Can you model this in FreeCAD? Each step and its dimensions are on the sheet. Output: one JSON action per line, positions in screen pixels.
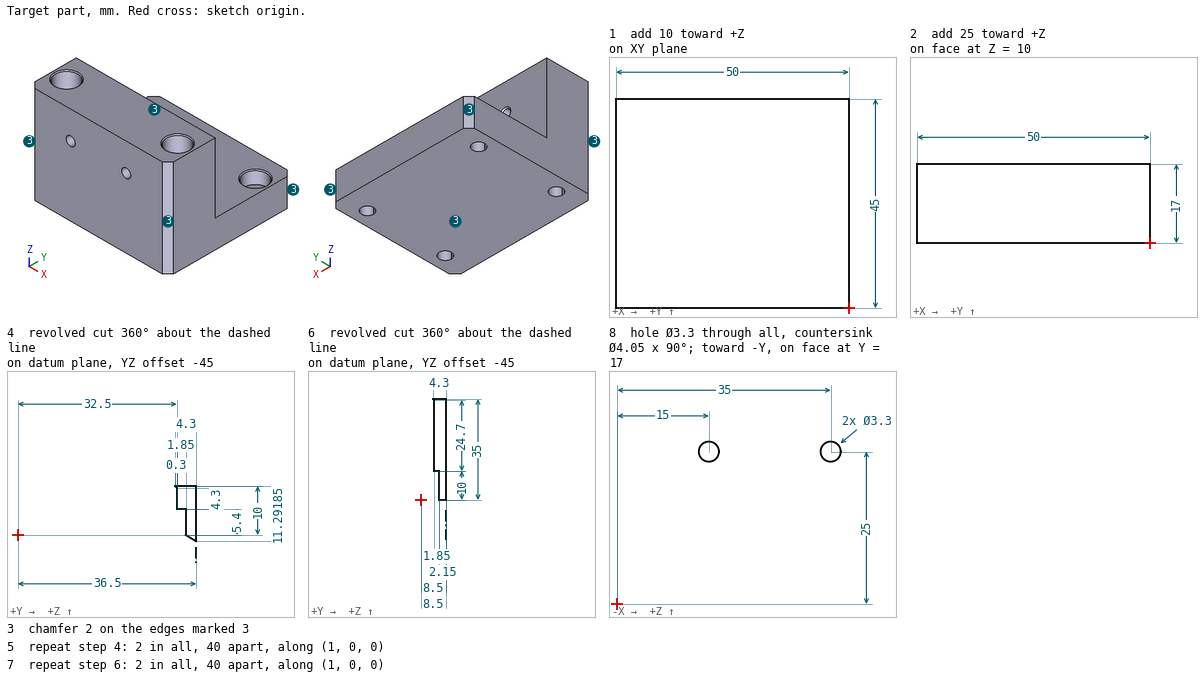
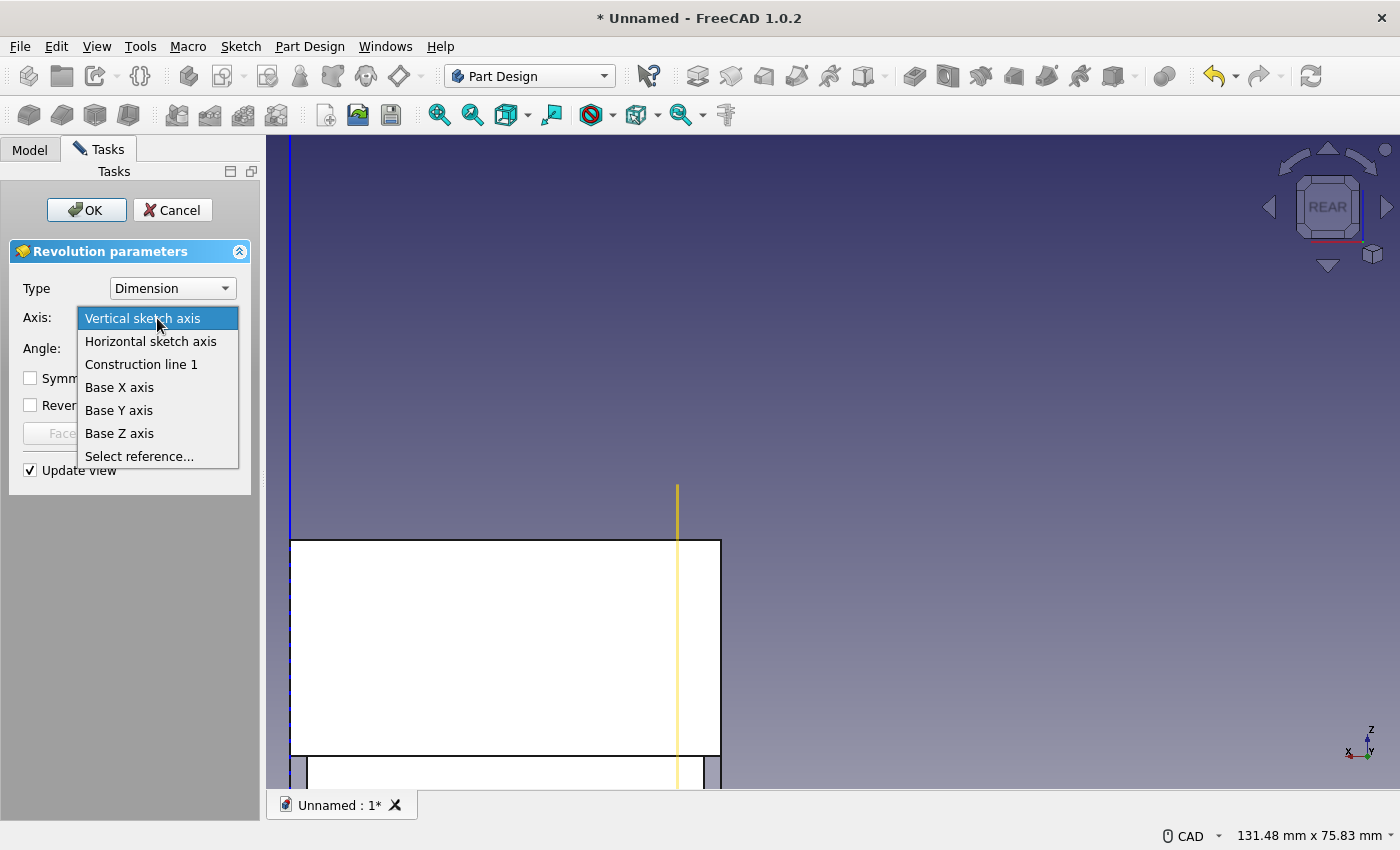
{"action": "left_click", "coordinate": [156, 364]}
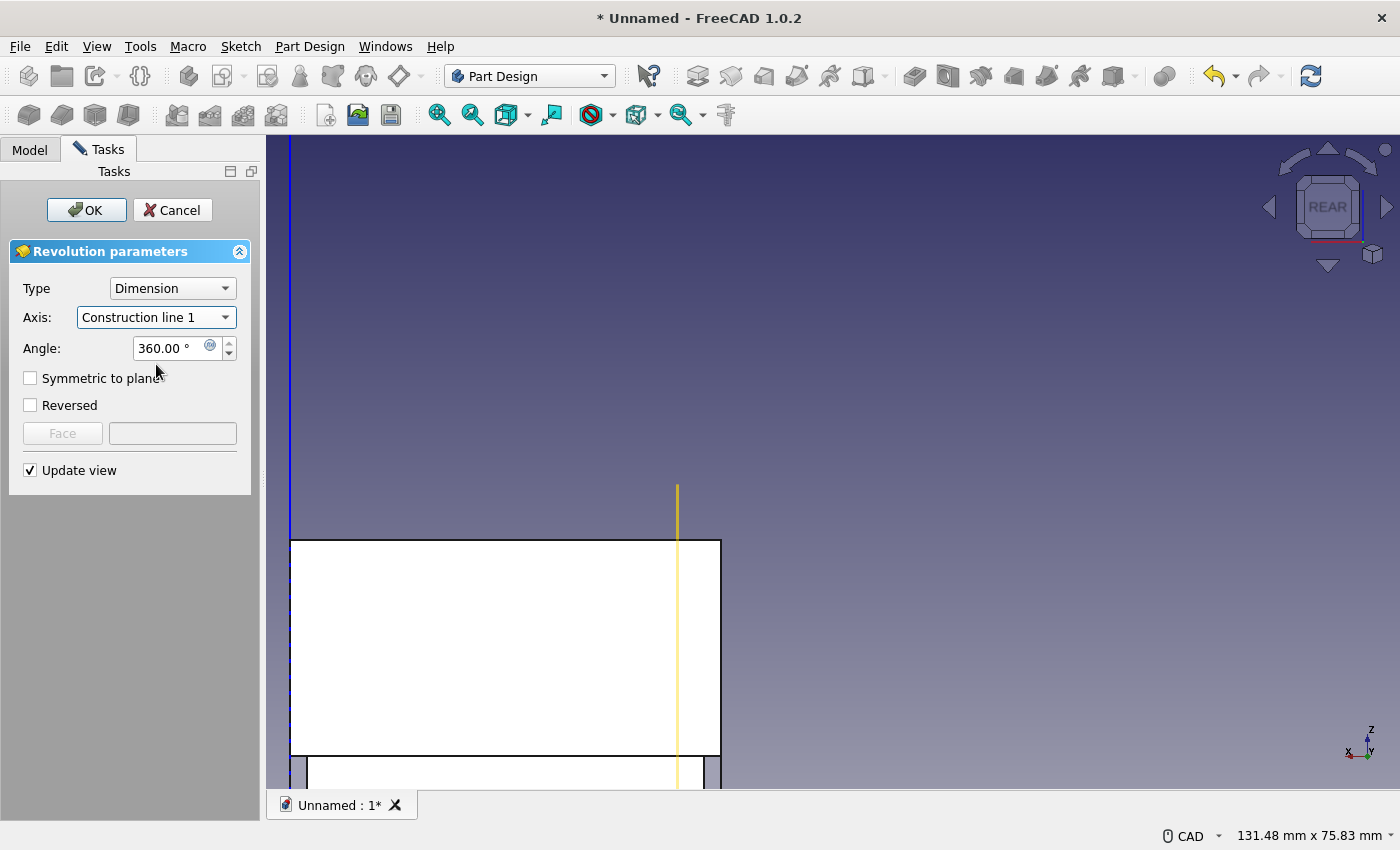
{"action": "left_click", "coordinate": [87, 210]}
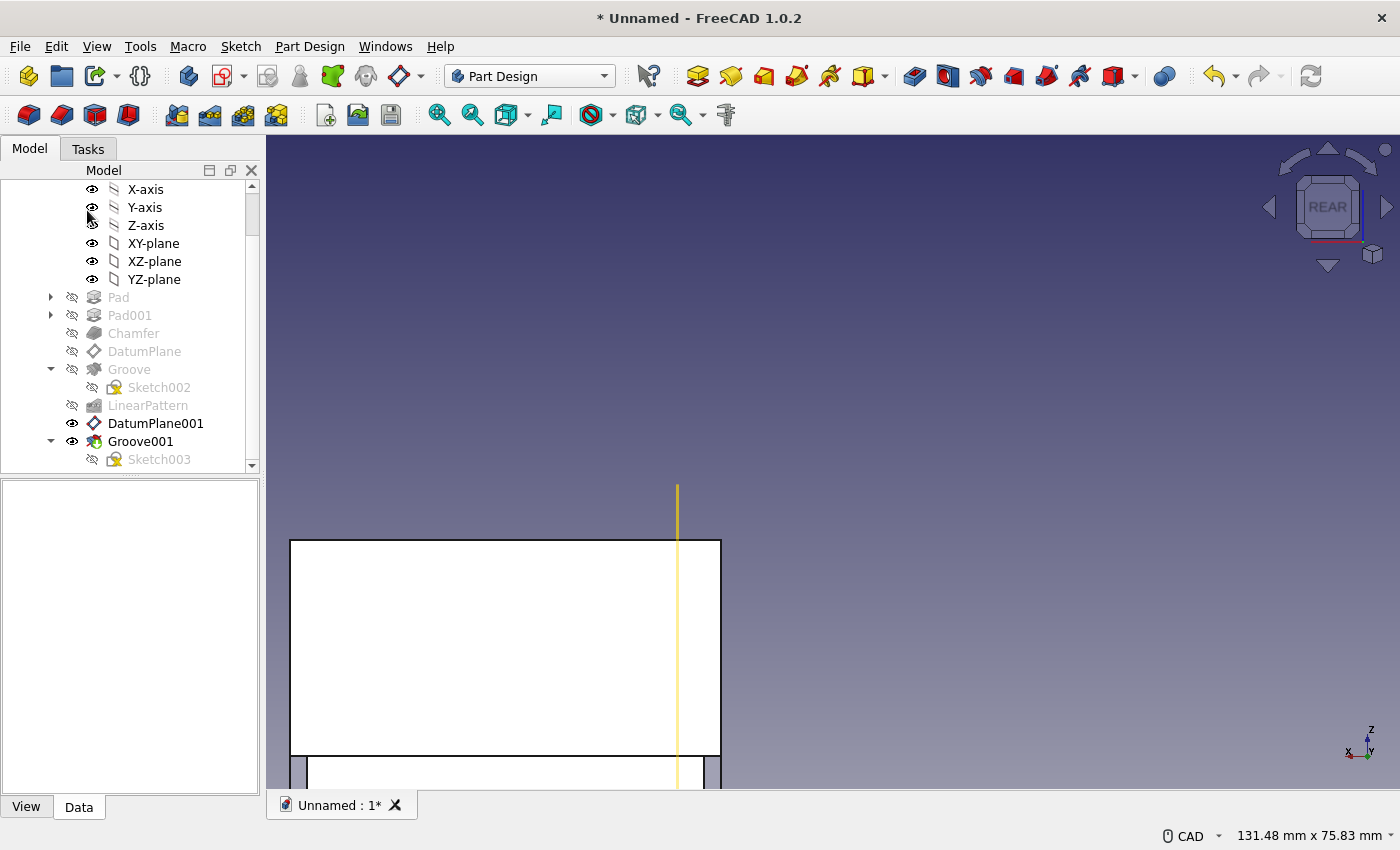
{"action": "left_click", "coordinate": [117, 423]}
{"action": "key", "text": "space"}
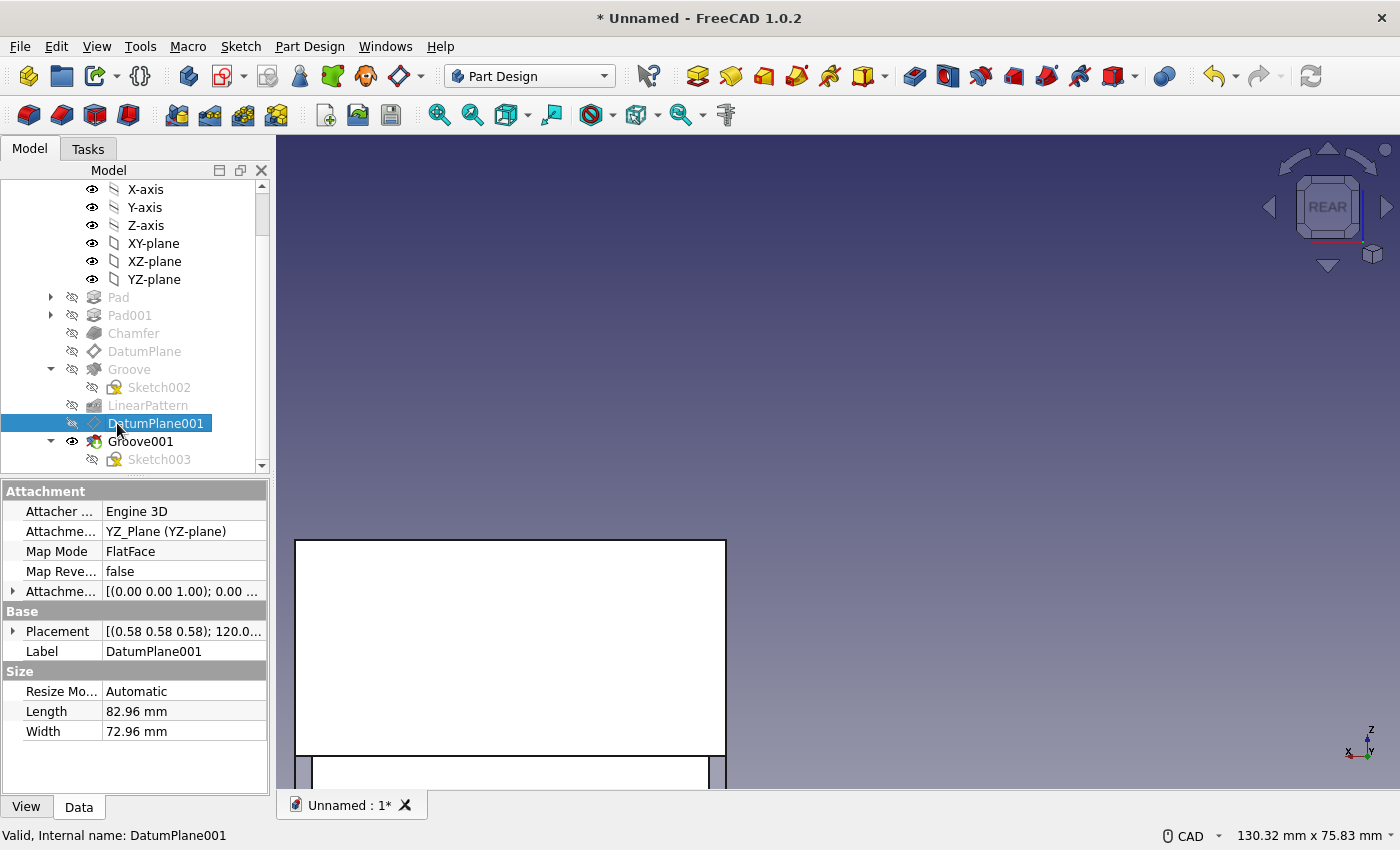
{"action": "left_click", "coordinate": [440, 116]}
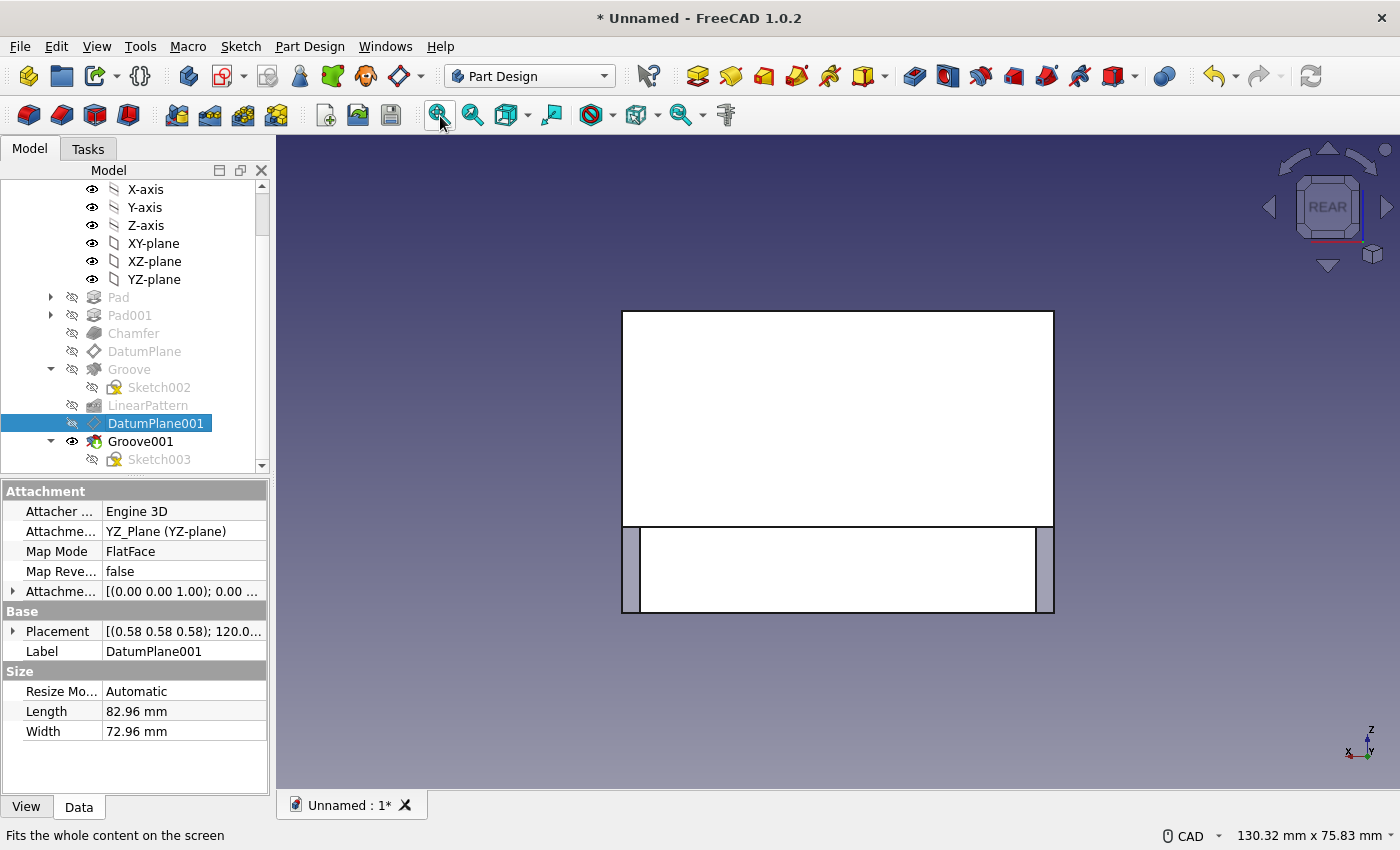
{"action": "left_click", "coordinate": [117, 441]}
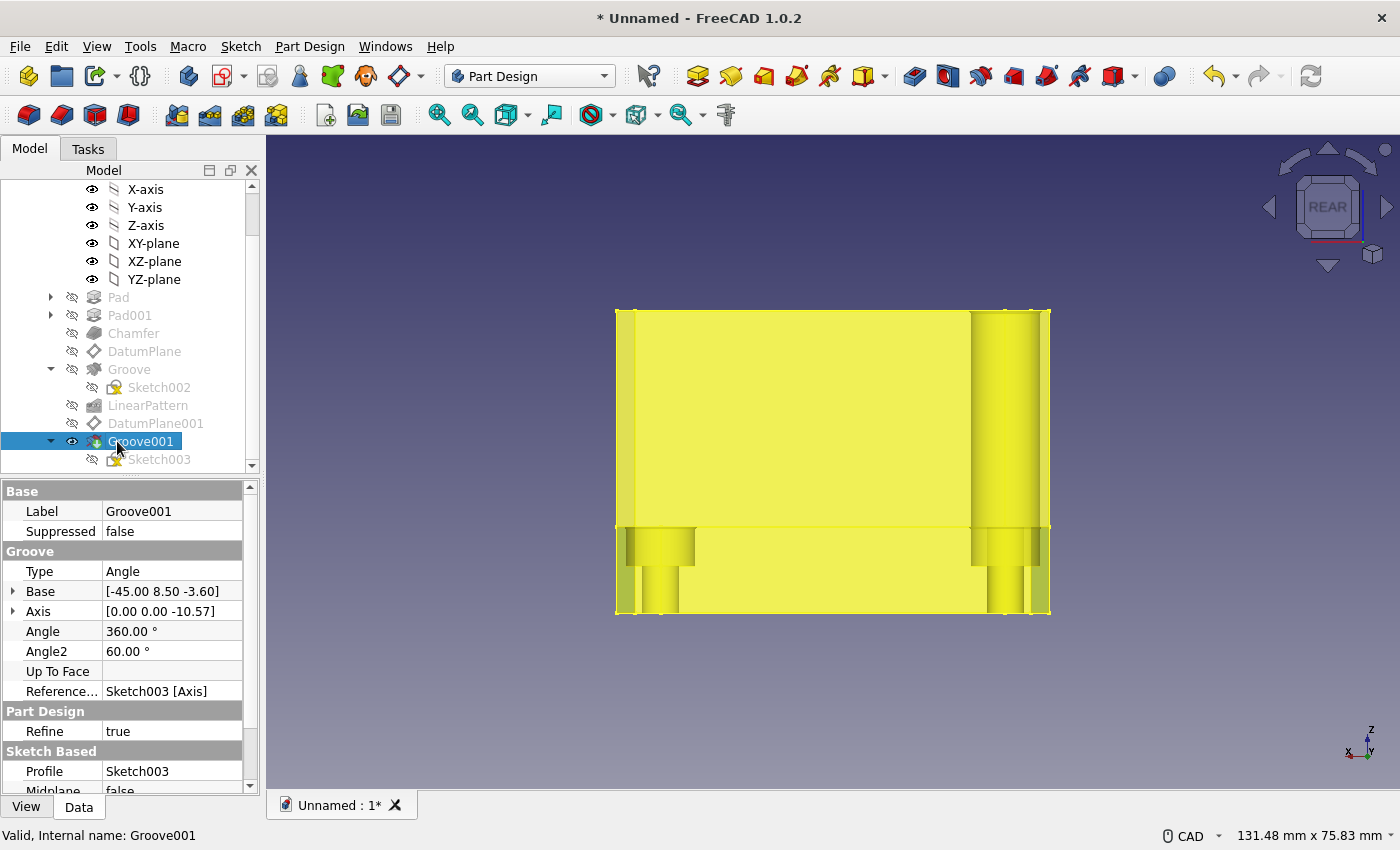
{"action": "left_click", "coordinate": [210, 116]}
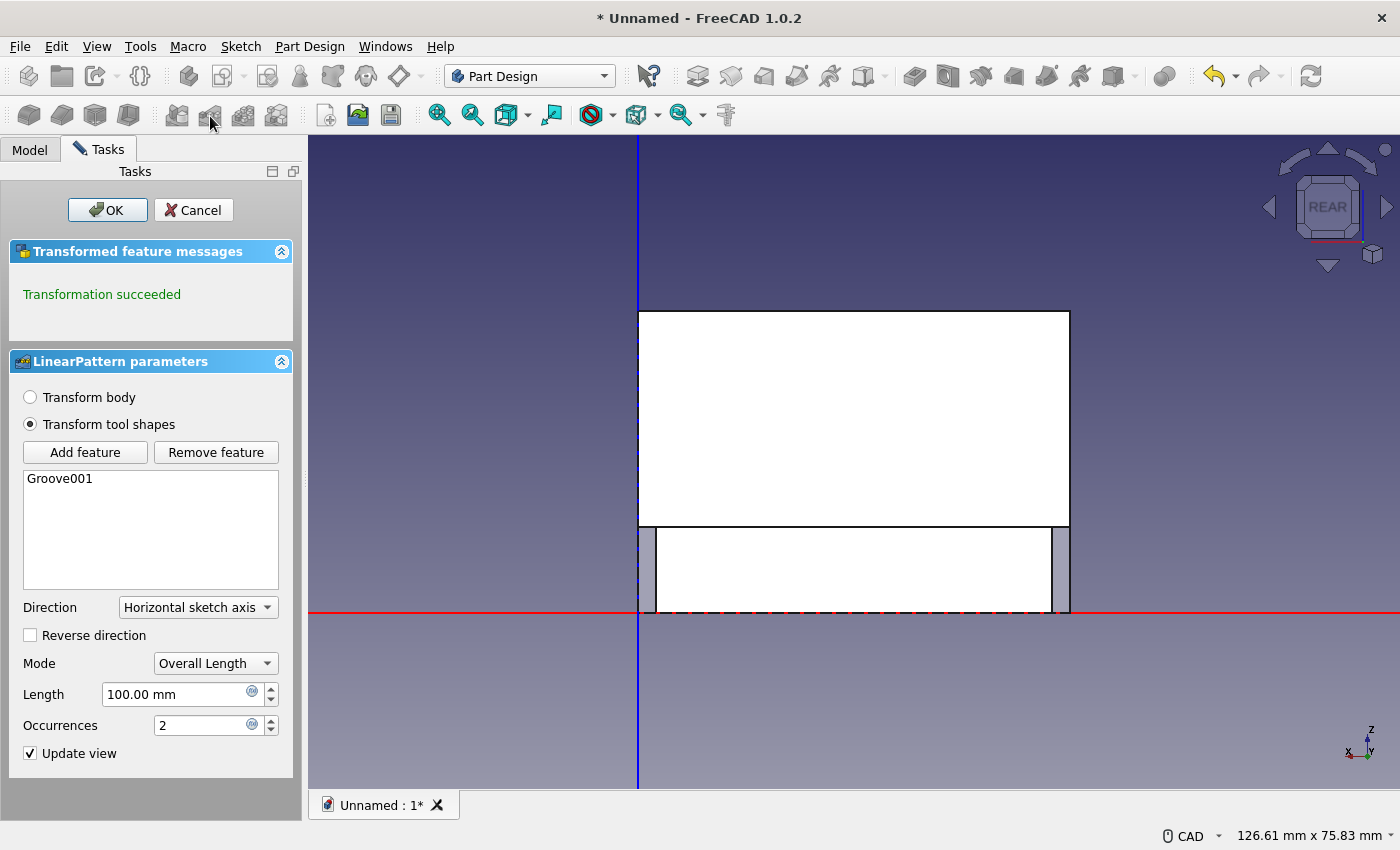
{"action": "left_click", "coordinate": [199, 608]}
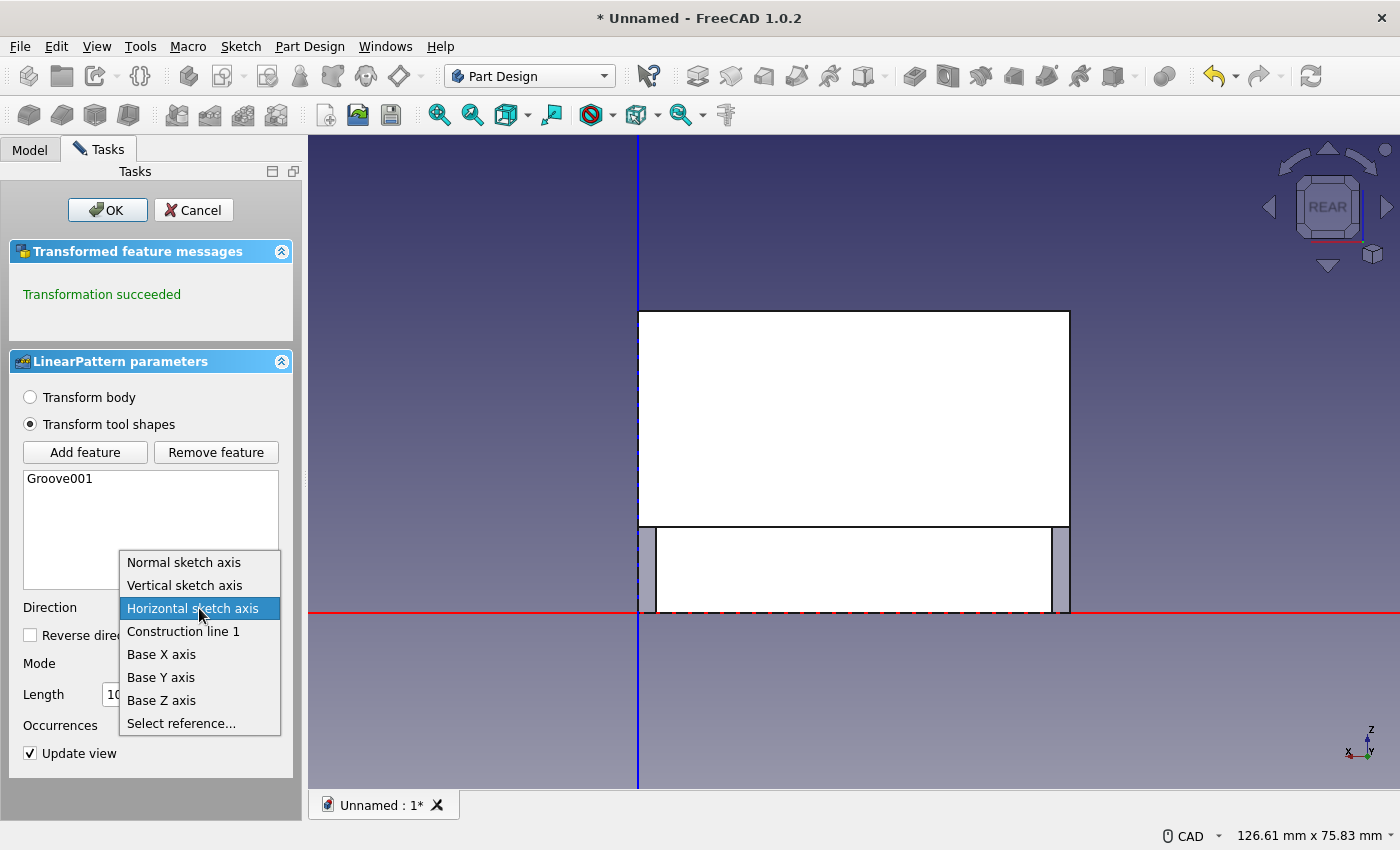
{"action": "left_click", "coordinate": [198, 654]}